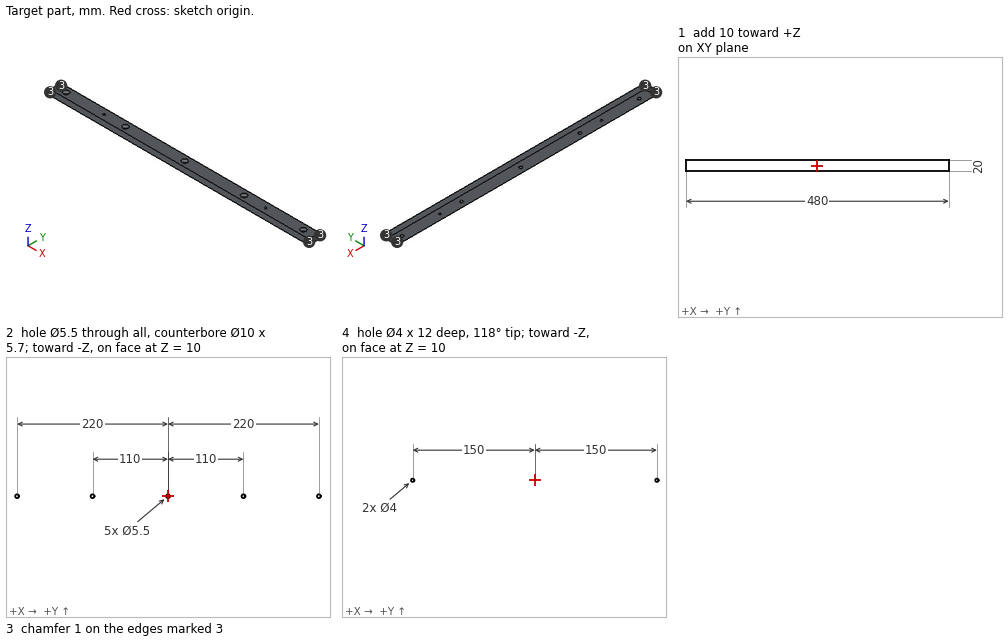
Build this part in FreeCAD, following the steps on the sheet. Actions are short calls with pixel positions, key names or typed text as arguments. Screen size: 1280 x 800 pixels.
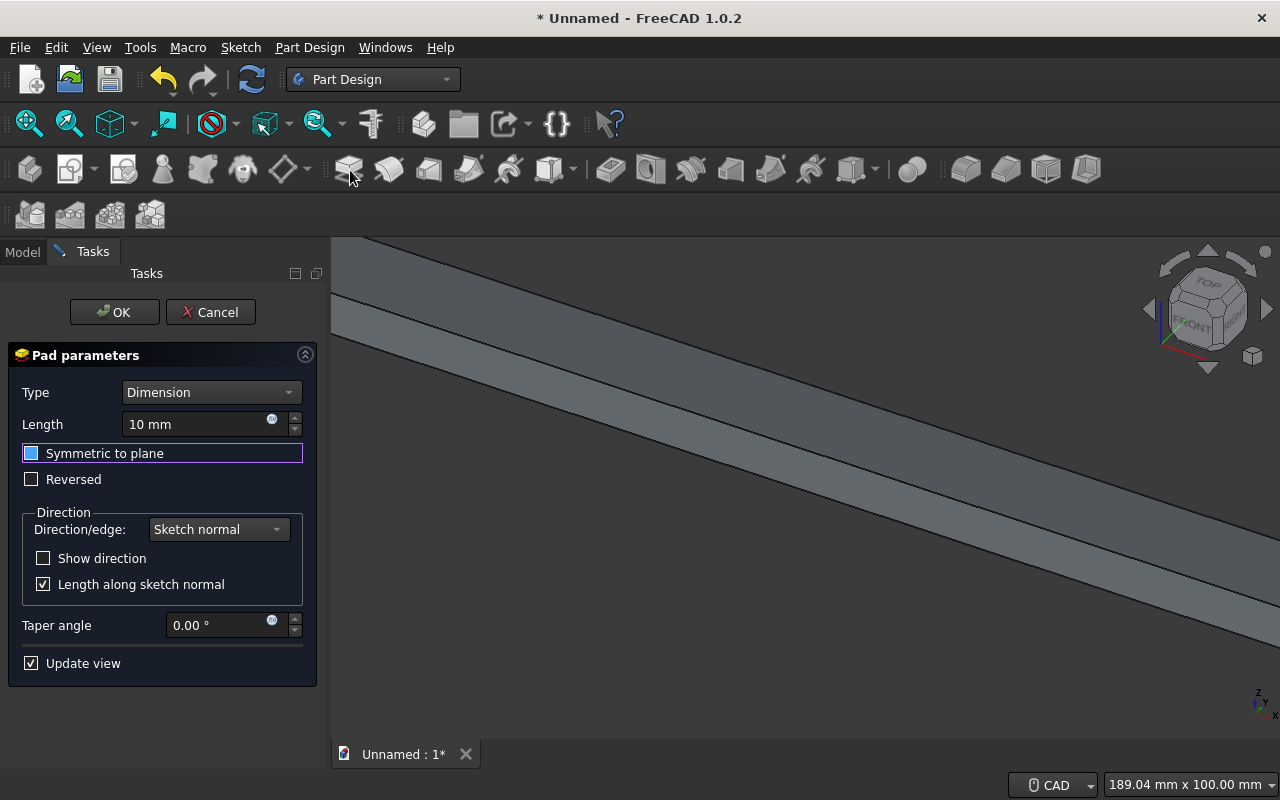
click(115, 312)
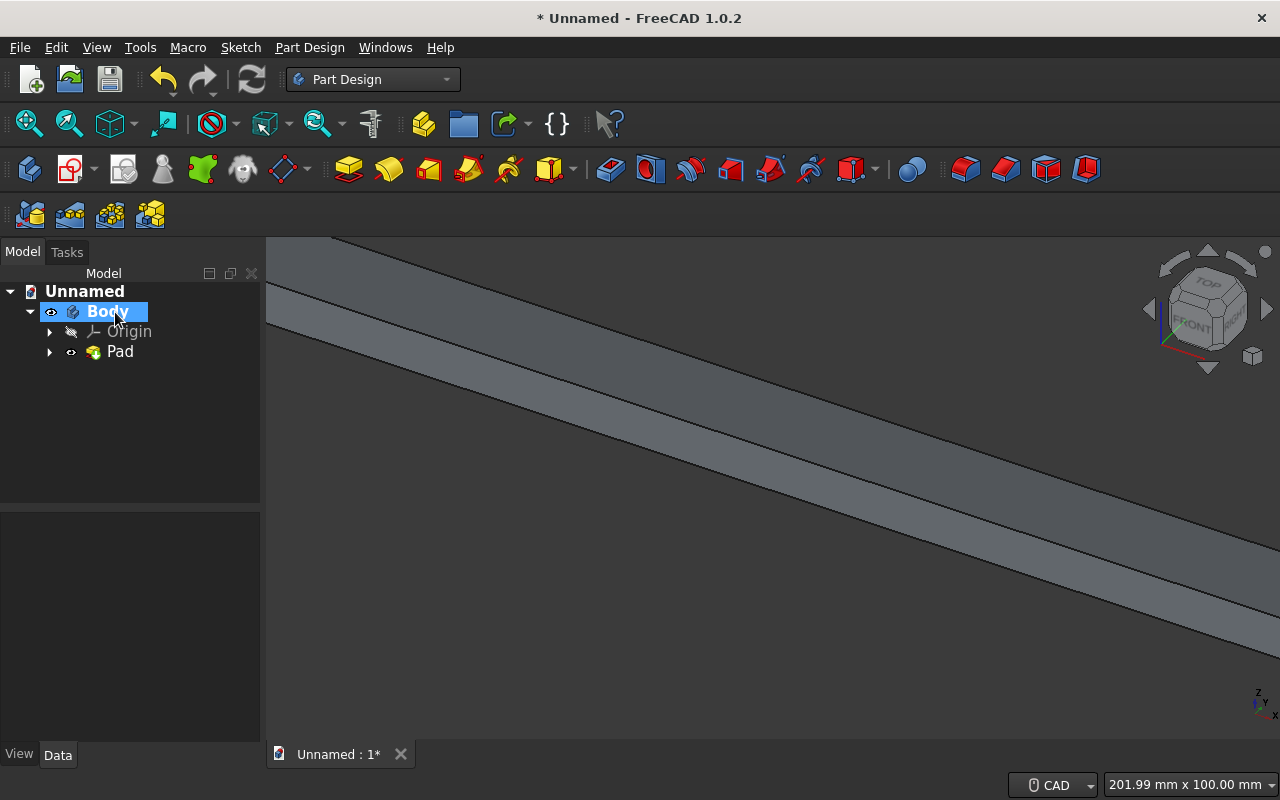
click(30, 124)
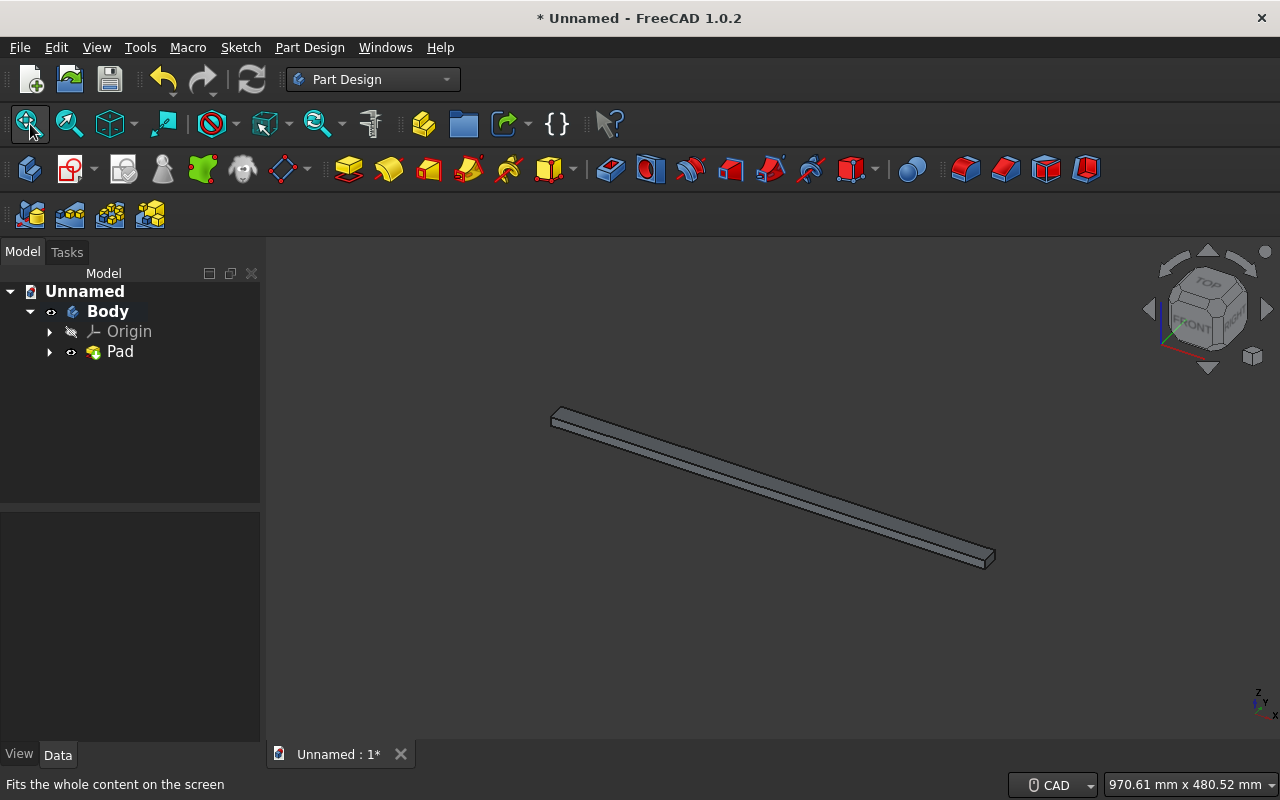
key(0)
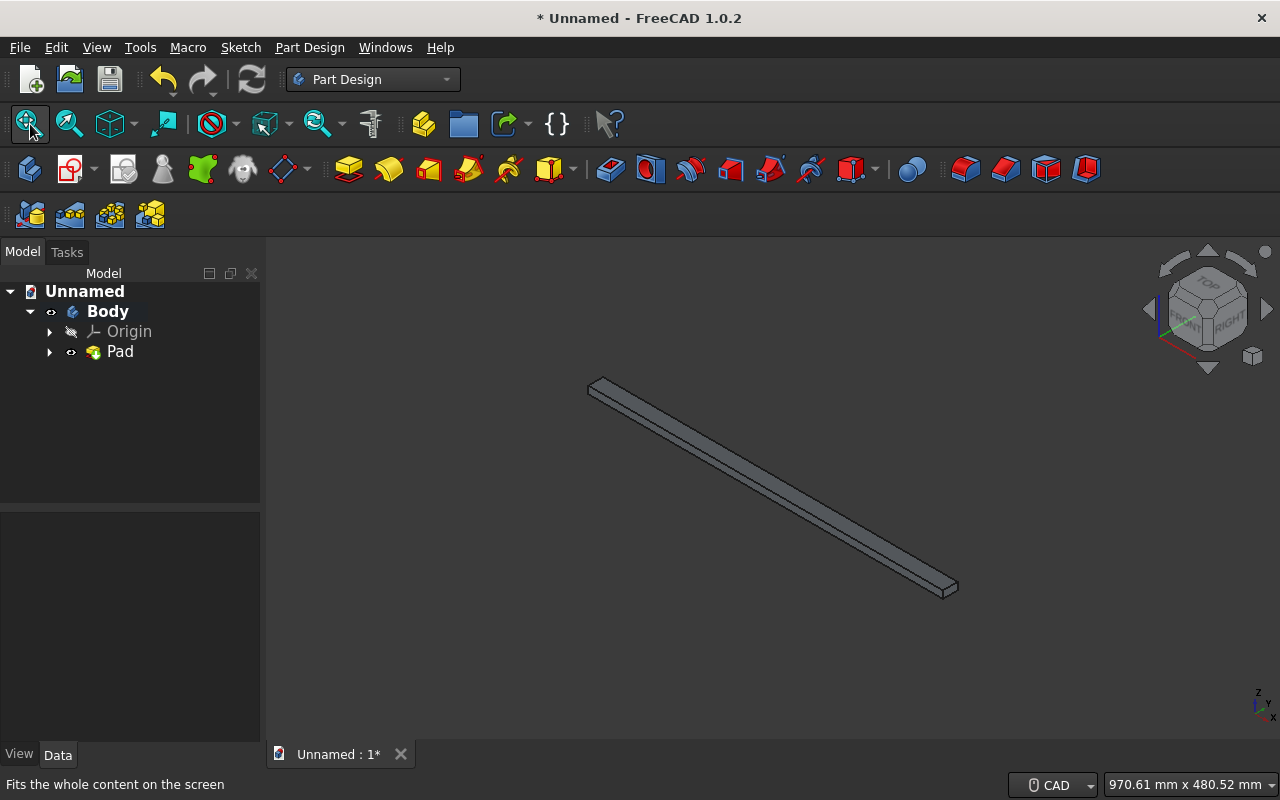
click(30, 124)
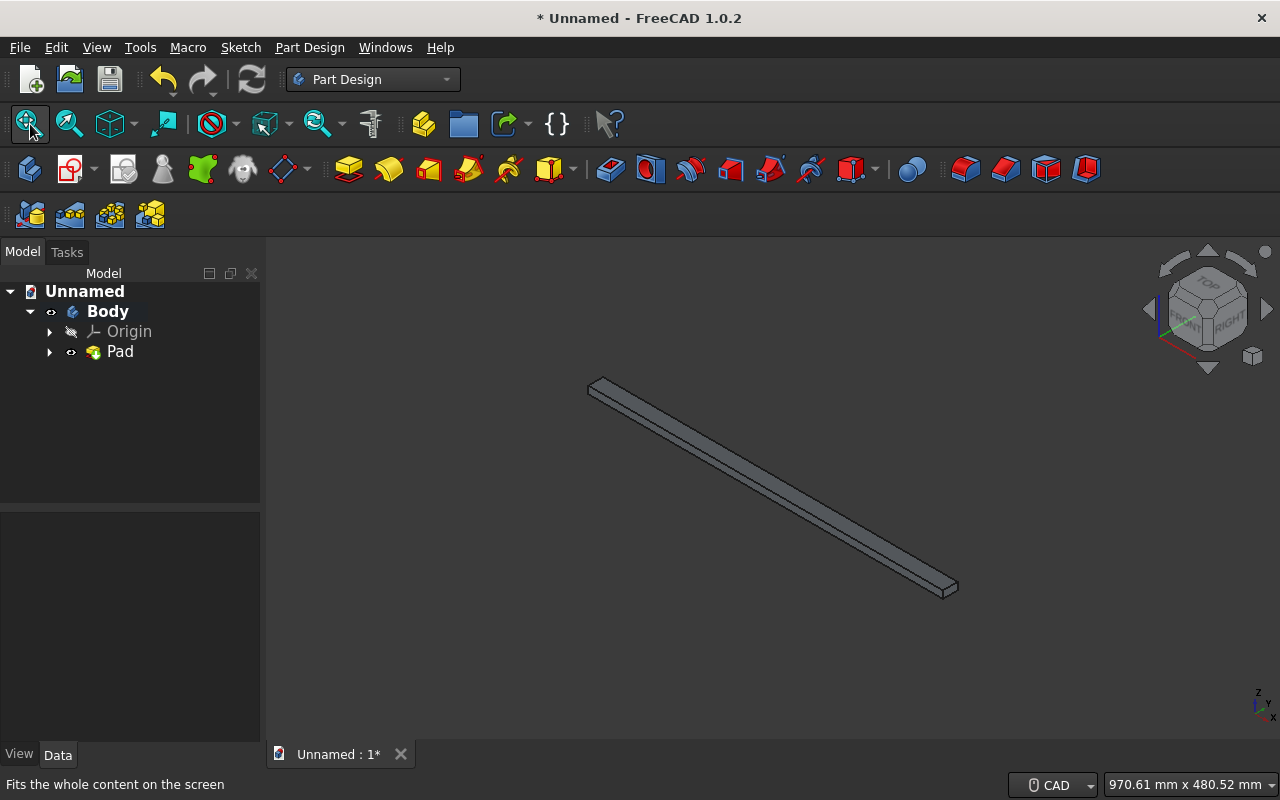
key(2)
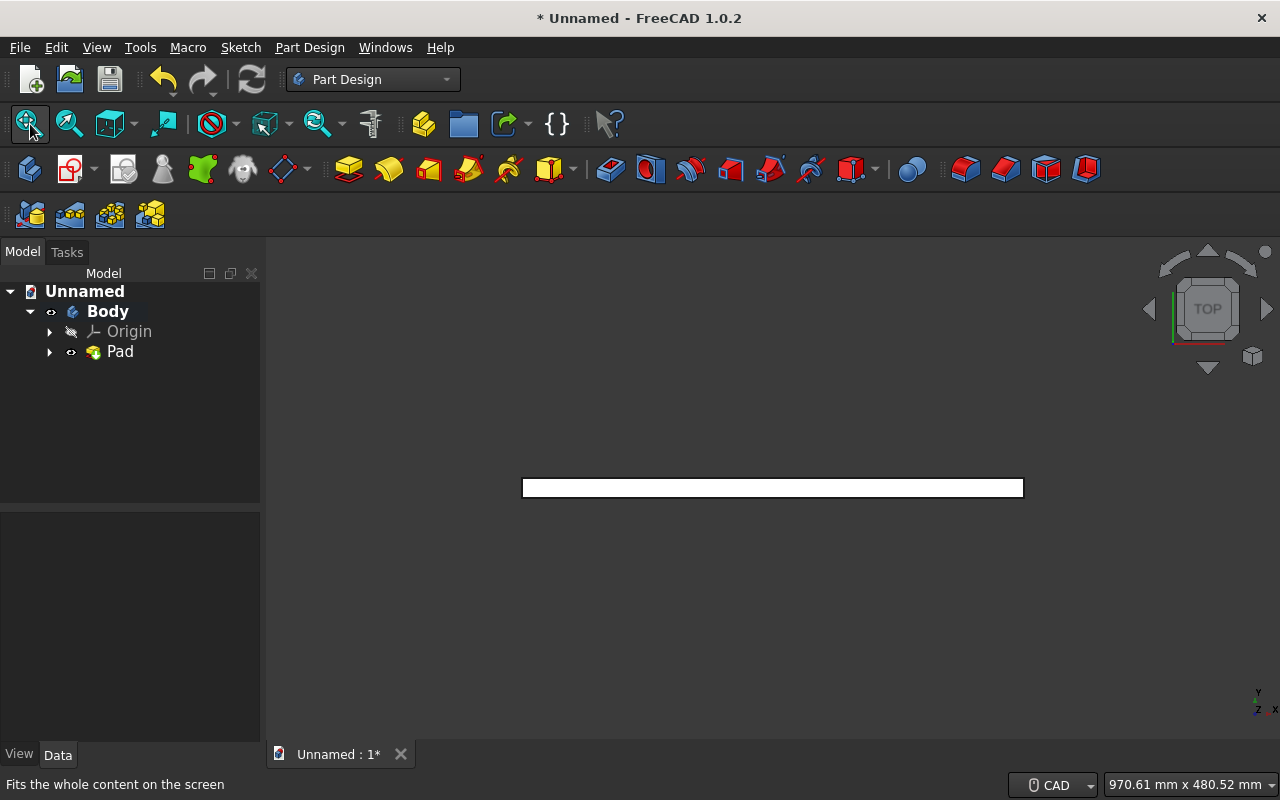
click(988, 487)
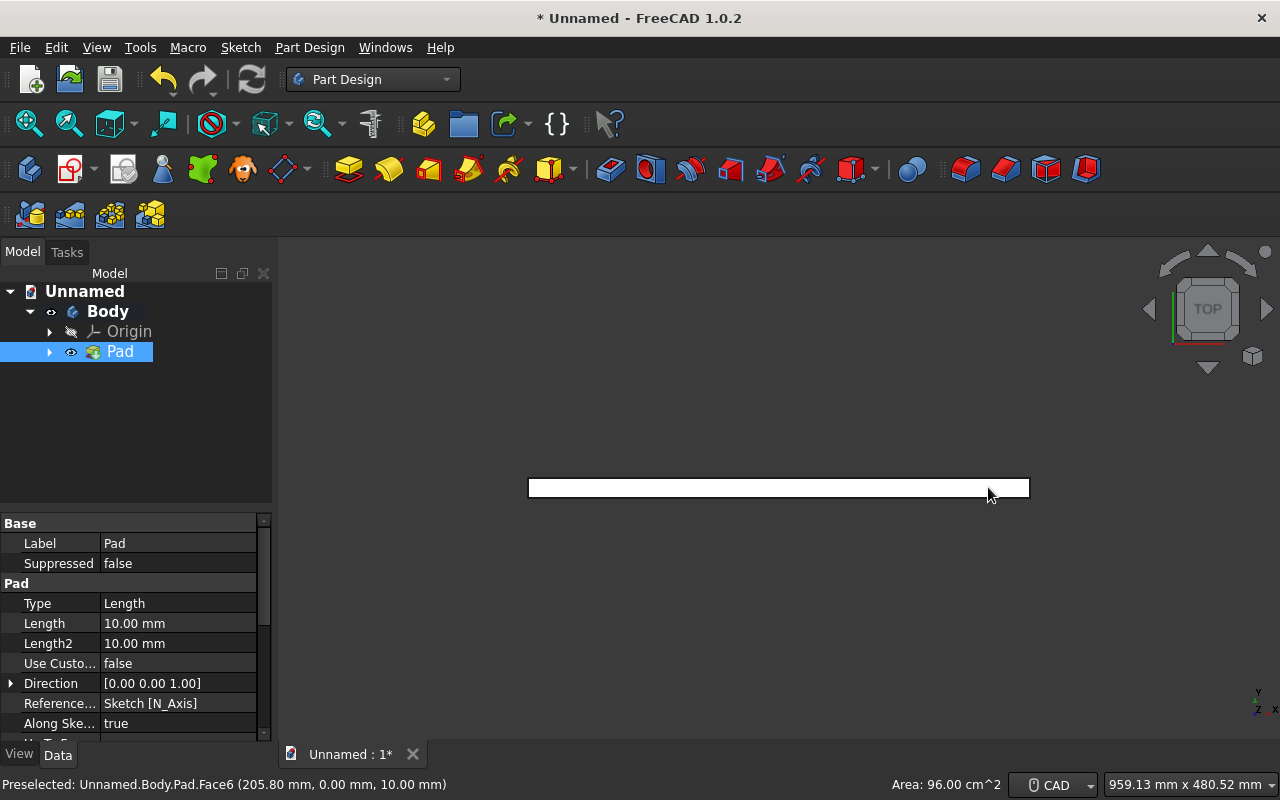
click(70, 170)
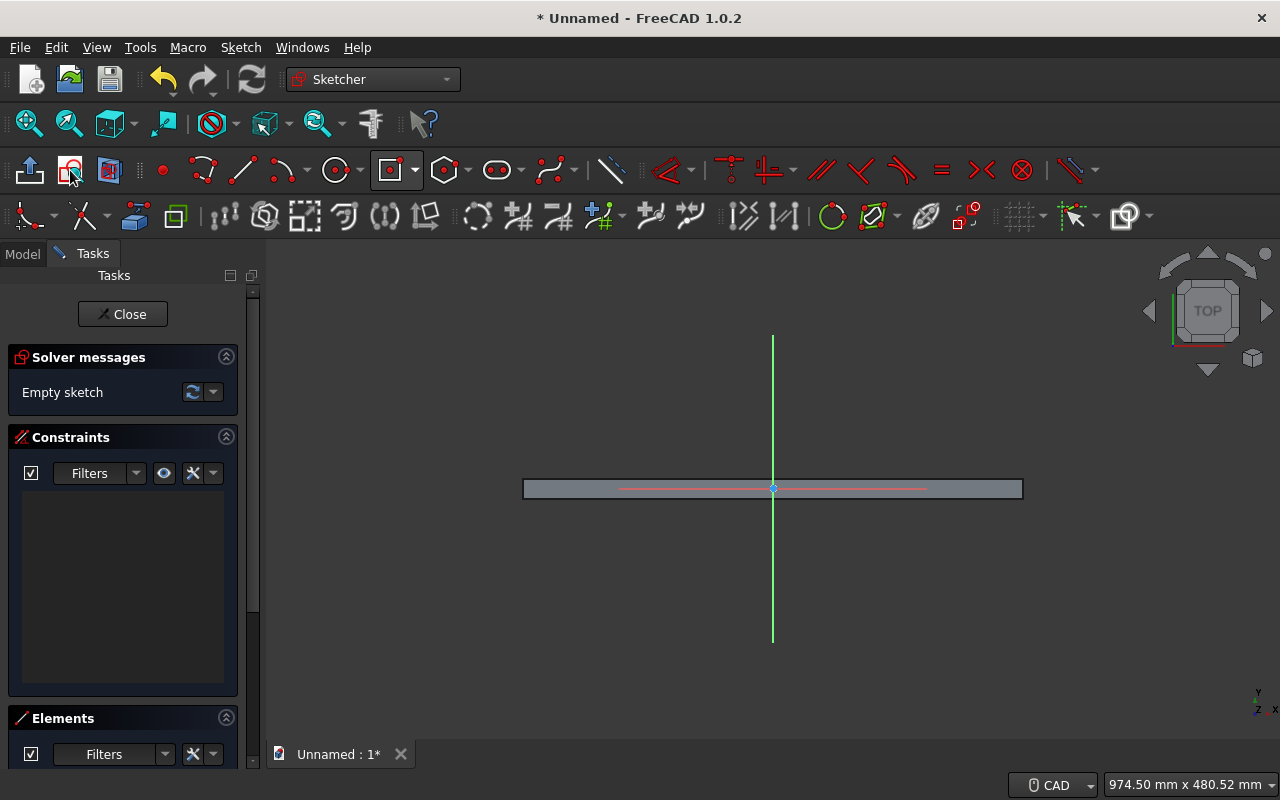
click(336, 170)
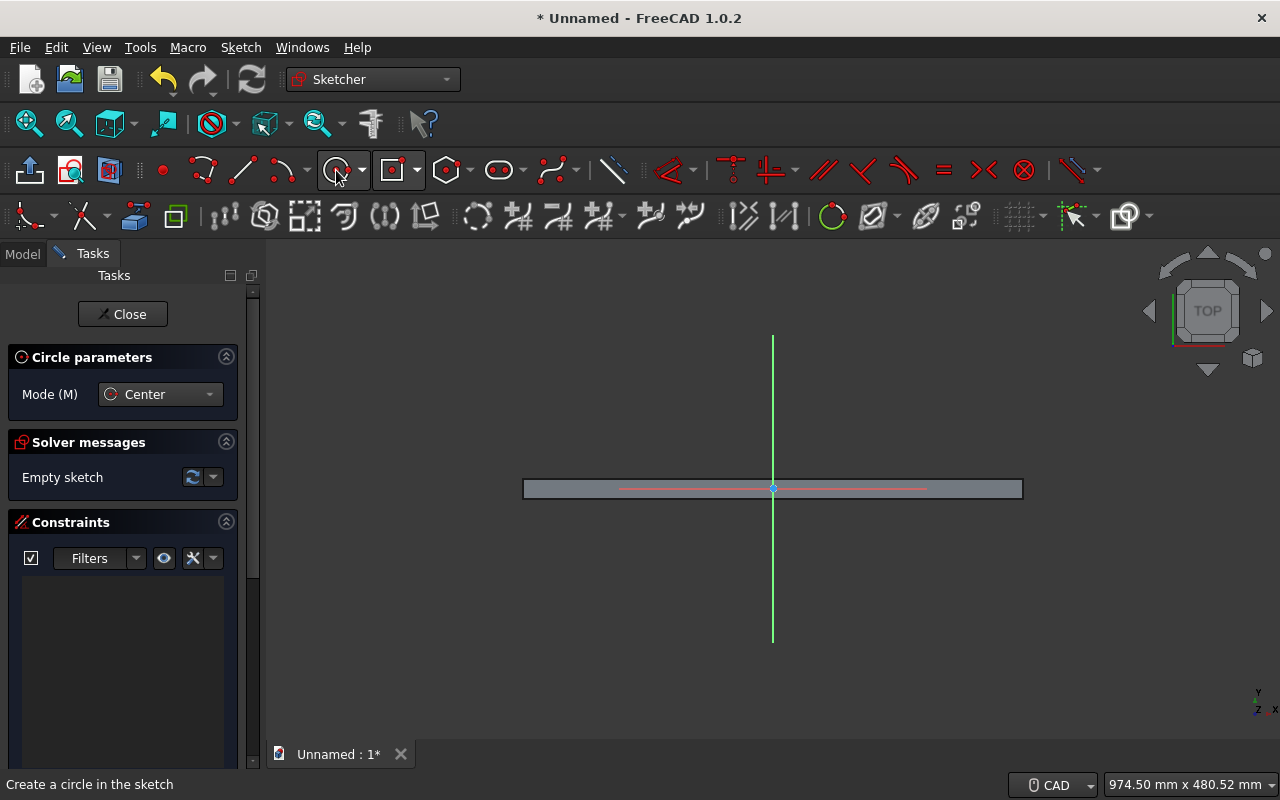
scroll(773, 489, up, 11)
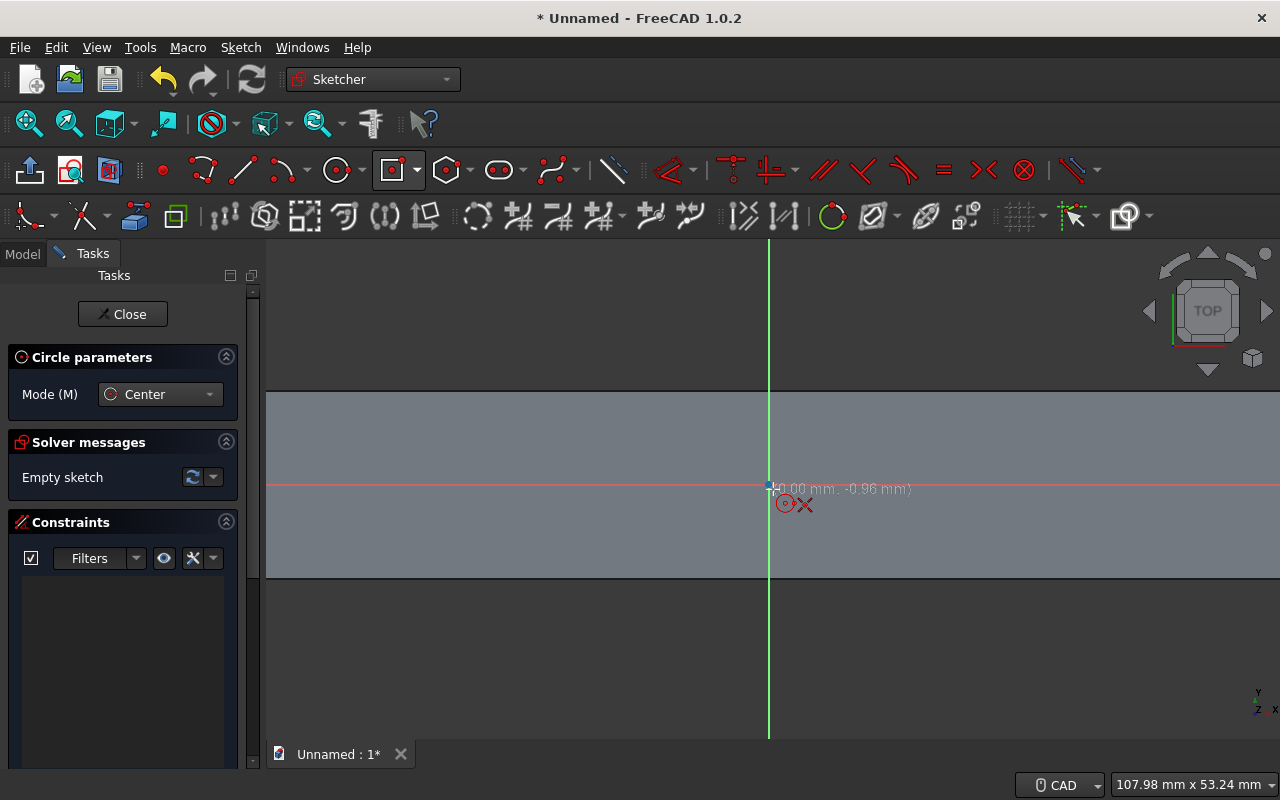
scroll(694, 490, down, 10)